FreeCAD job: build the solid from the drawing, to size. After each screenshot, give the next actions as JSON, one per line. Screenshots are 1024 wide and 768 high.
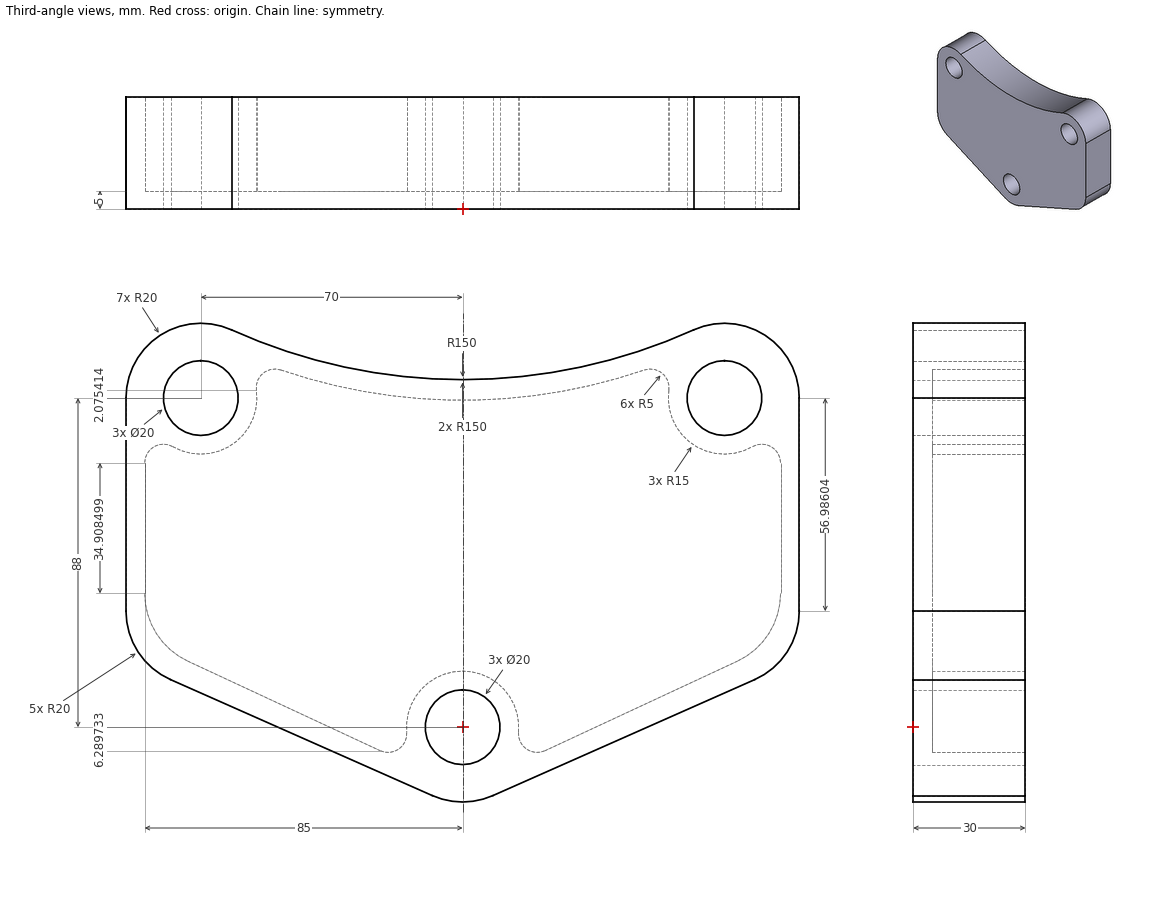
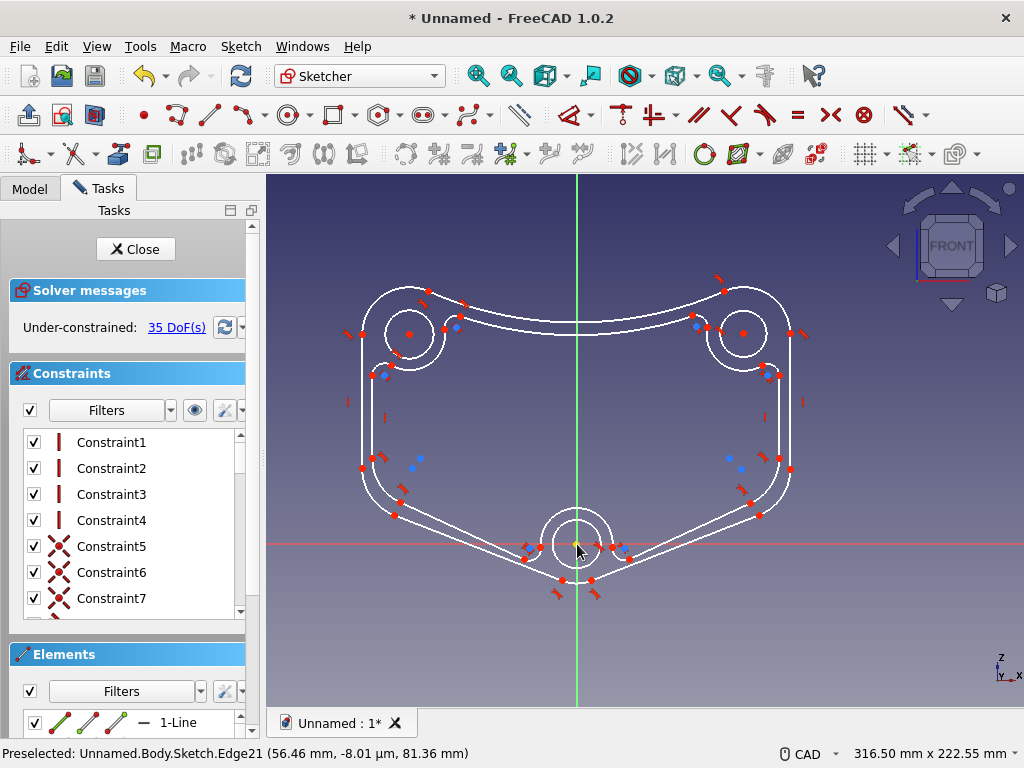
{"action": "left_click", "coordinate": [774, 506]}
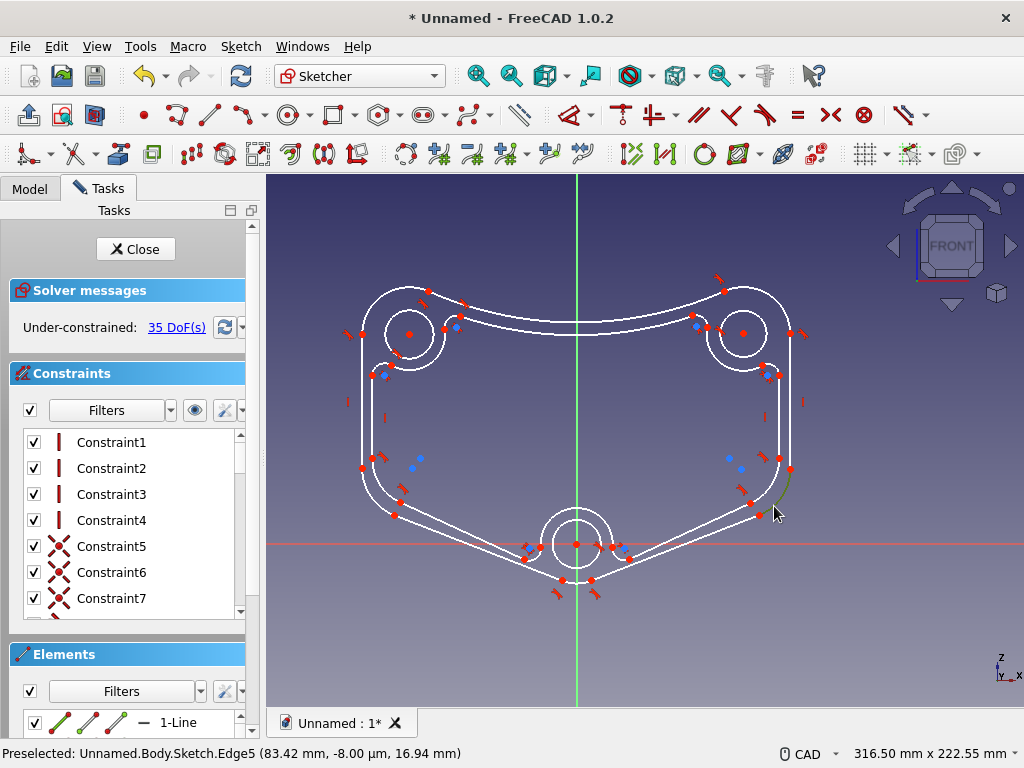
{"action": "left_click", "coordinate": [577, 584]}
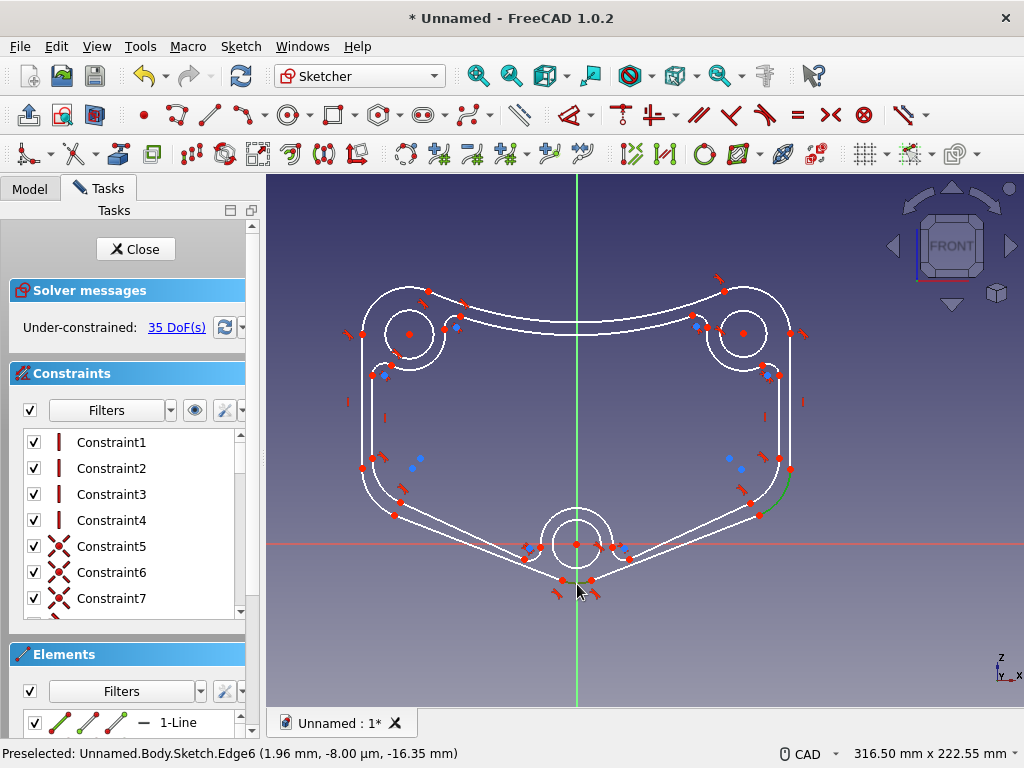
{"action": "left_click", "coordinate": [365, 486]}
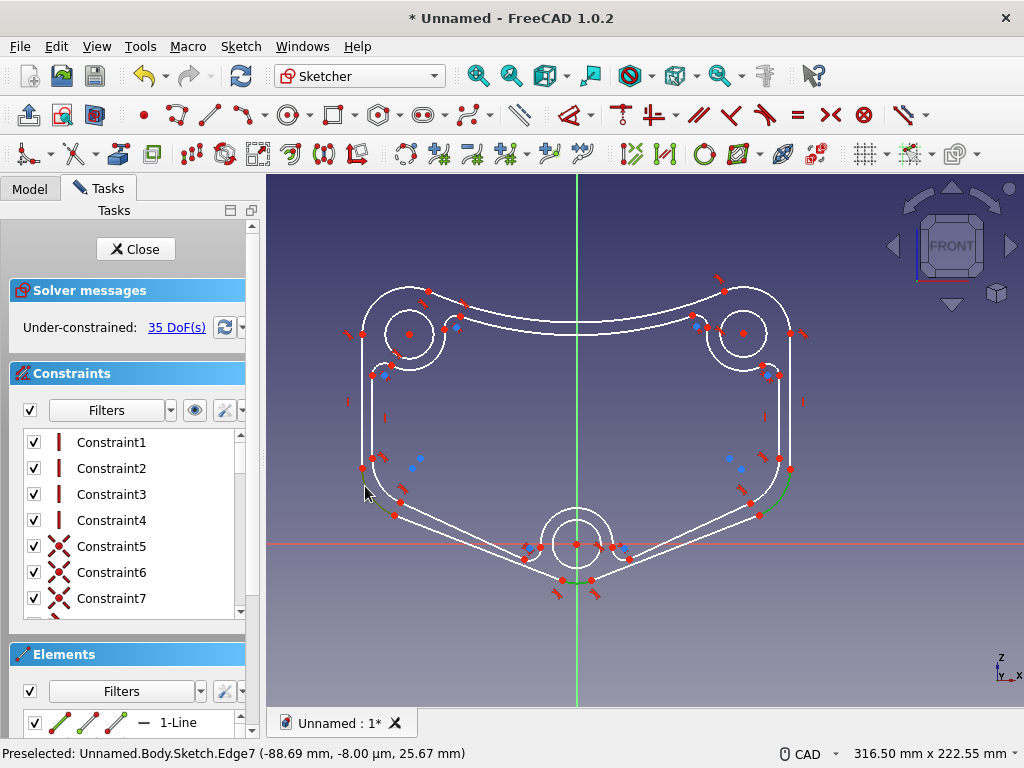
{"action": "left_click", "coordinate": [401, 288]}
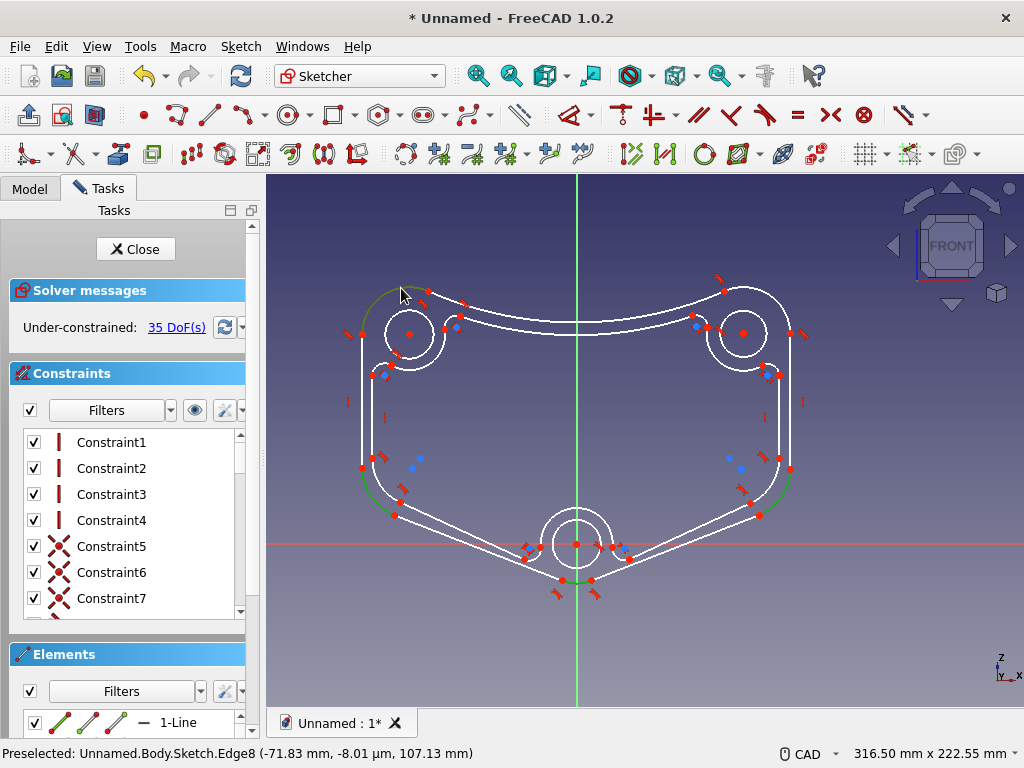
{"action": "left_click", "coordinate": [782, 308]}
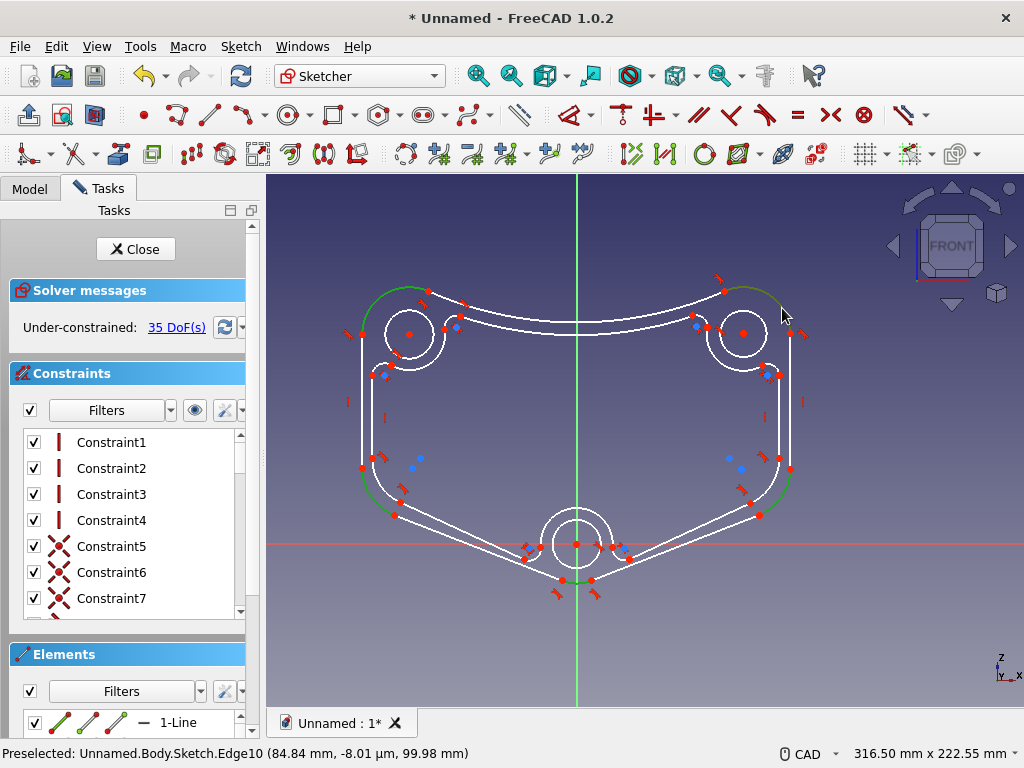
{"action": "left_click", "coordinate": [375, 475]}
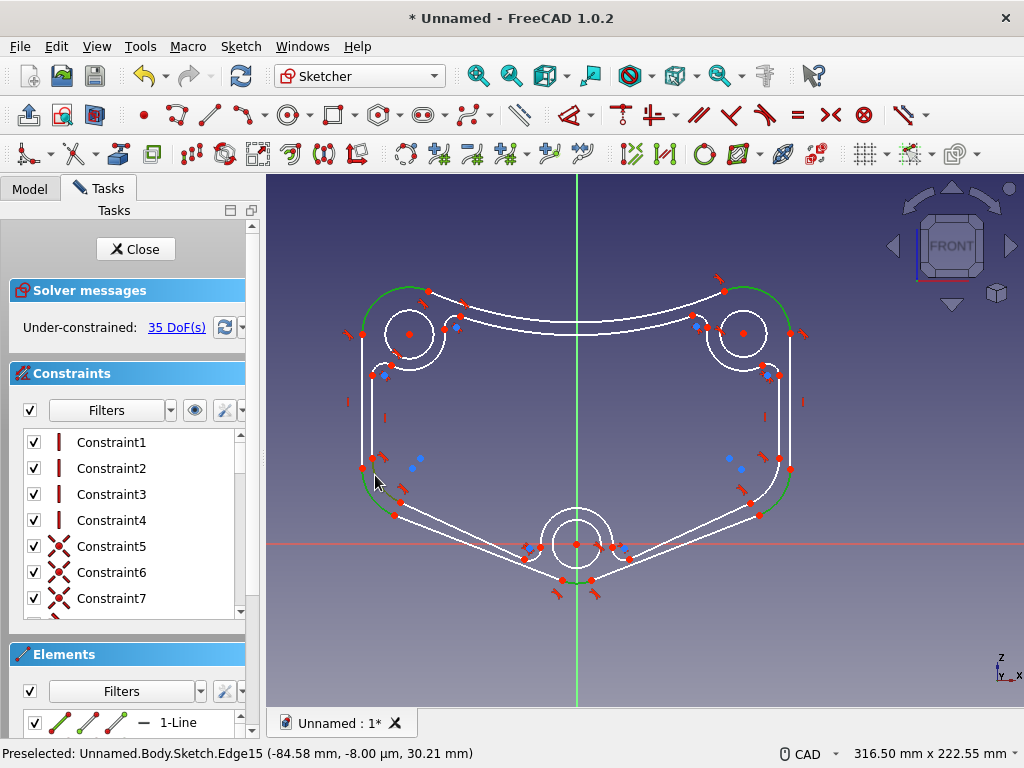
{"action": "left_click", "coordinate": [764, 494]}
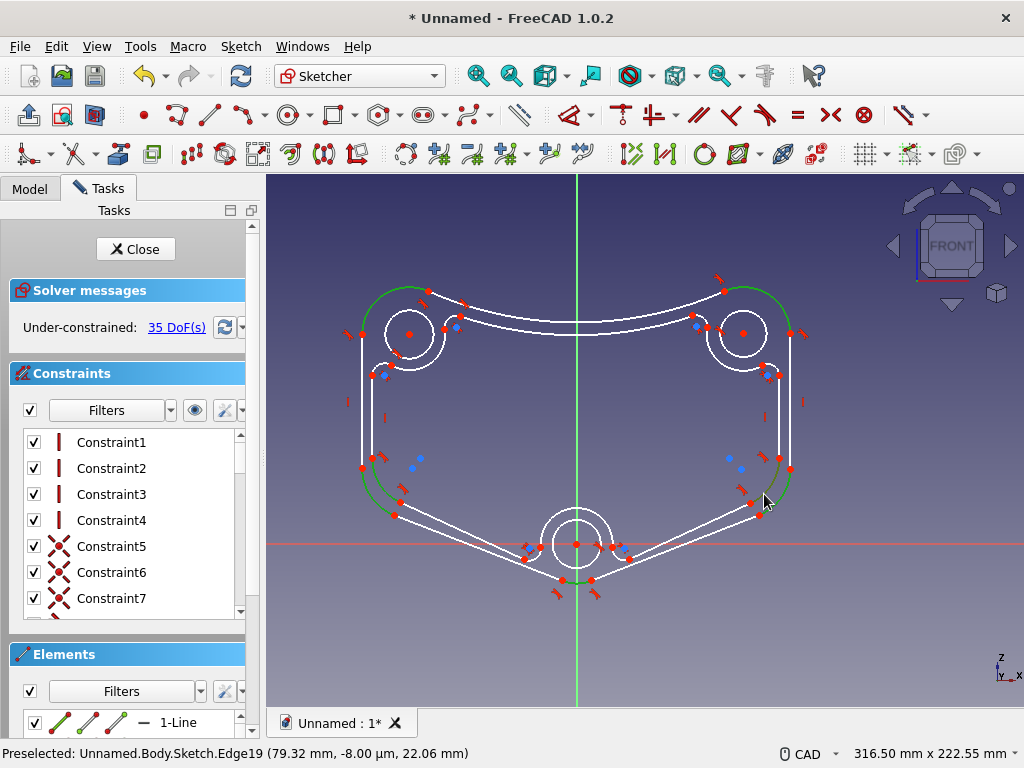
{"action": "key", "text": "e"}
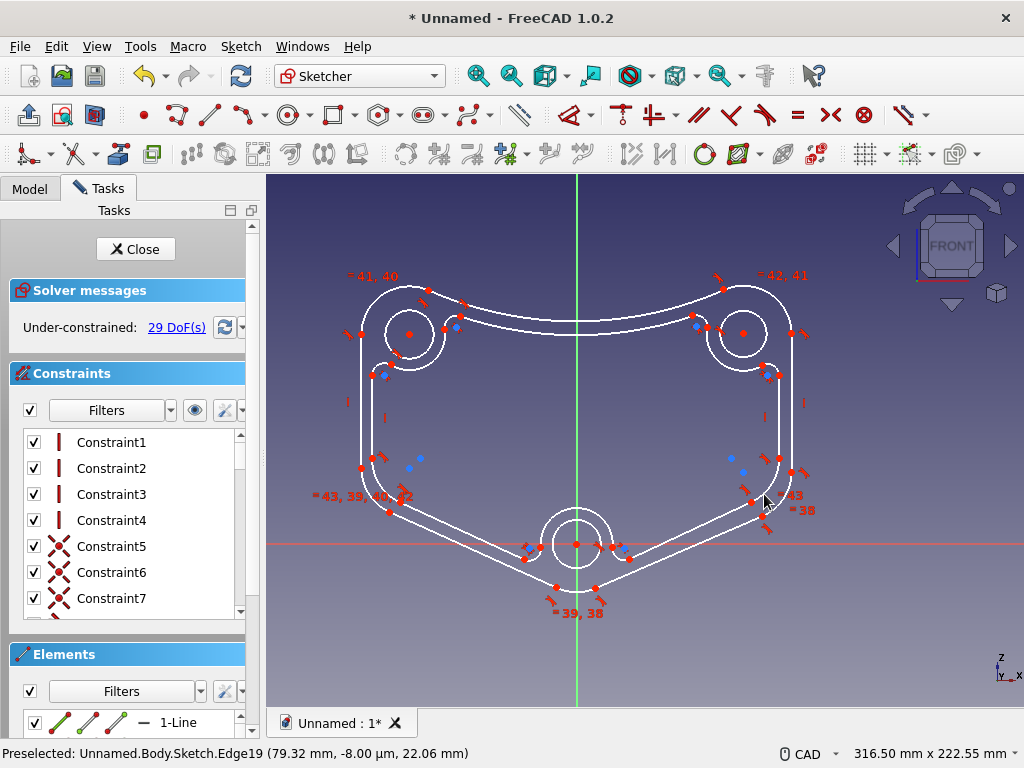
{"action": "left_click", "coordinate": [536, 558]}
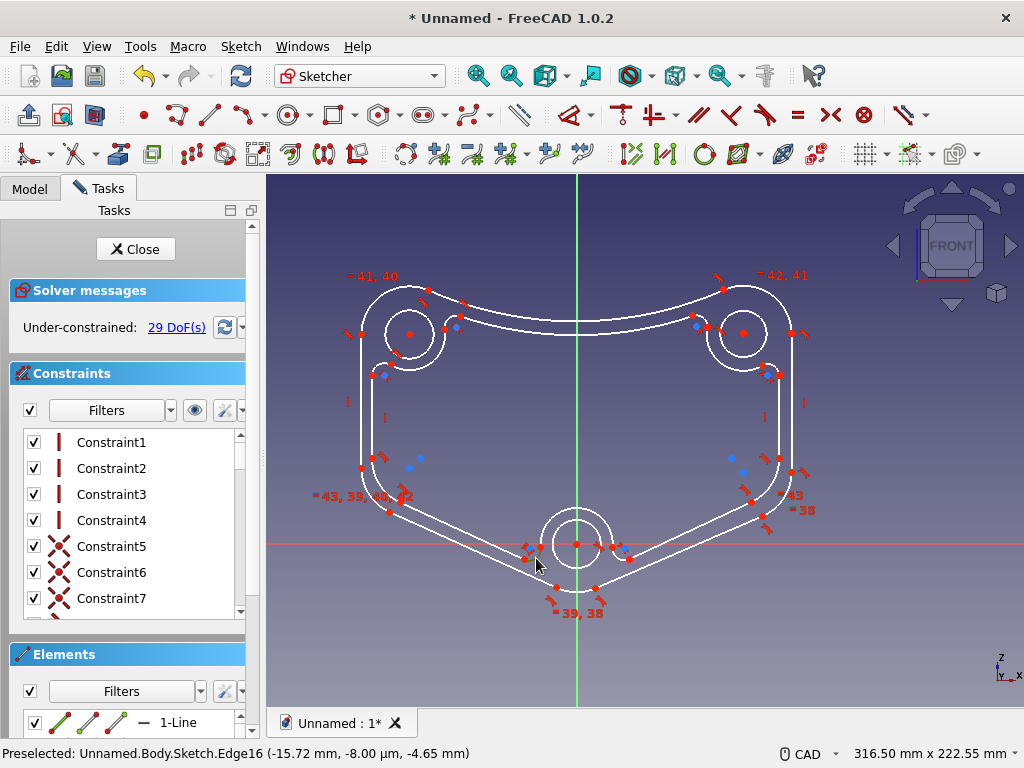
{"action": "left_click", "coordinate": [618, 558]}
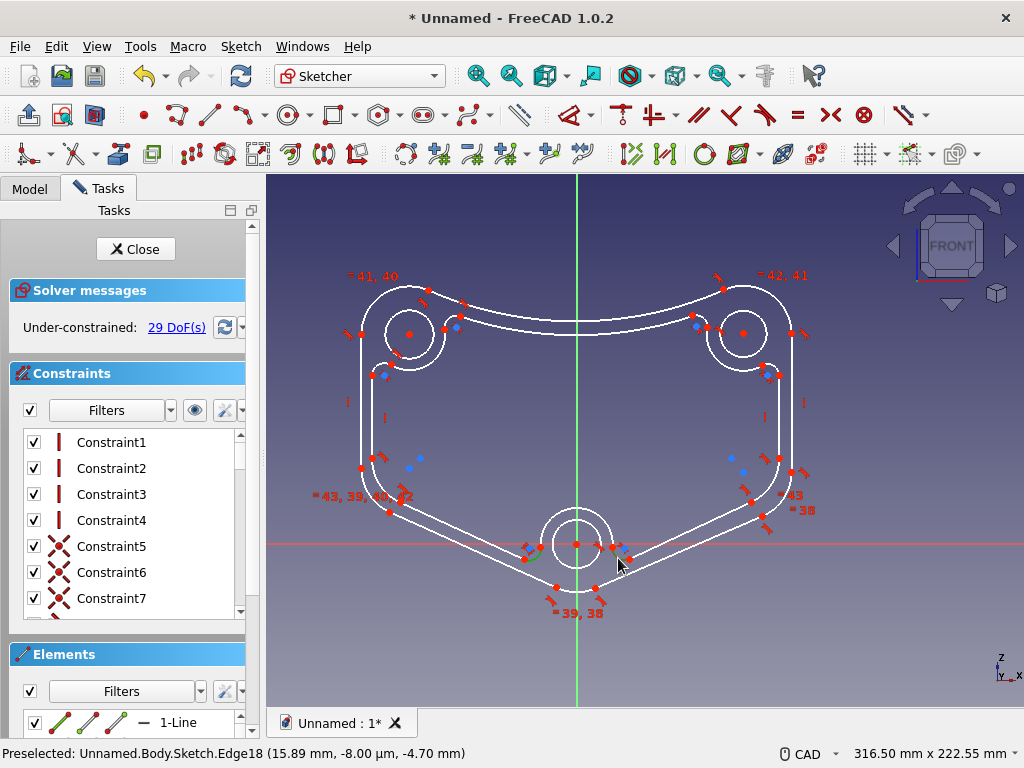
{"action": "scroll", "coordinate": [773, 366], "scroll_direction": "up", "scroll_amount": 2}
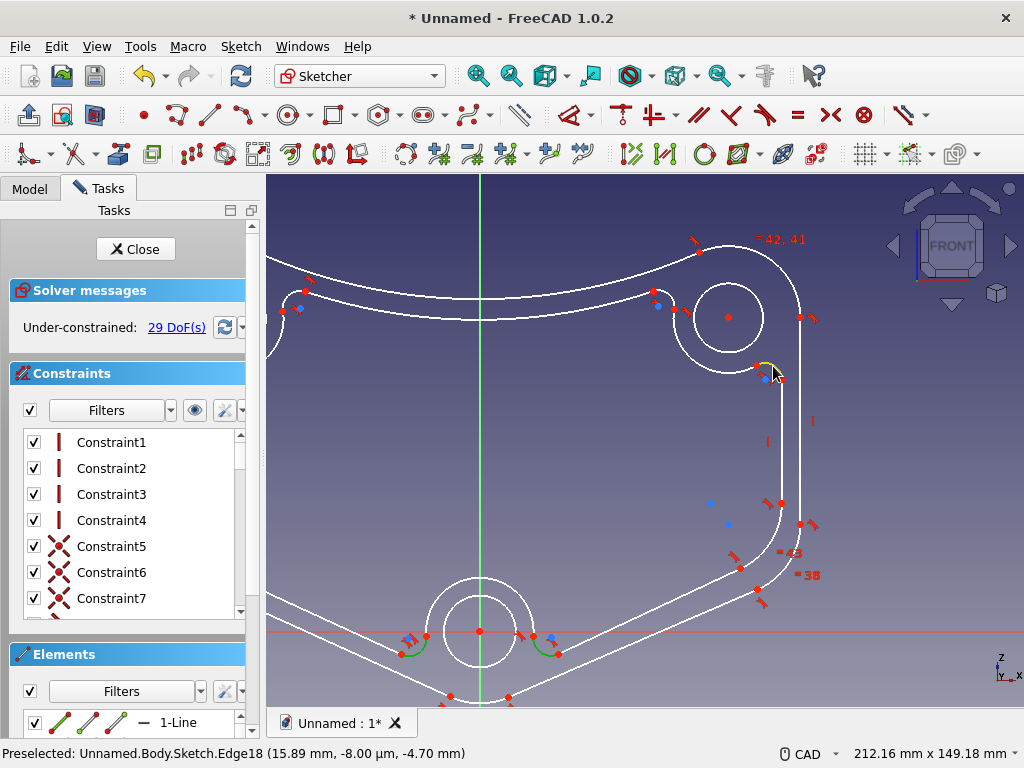
{"action": "left_click", "coordinate": [773, 365]}